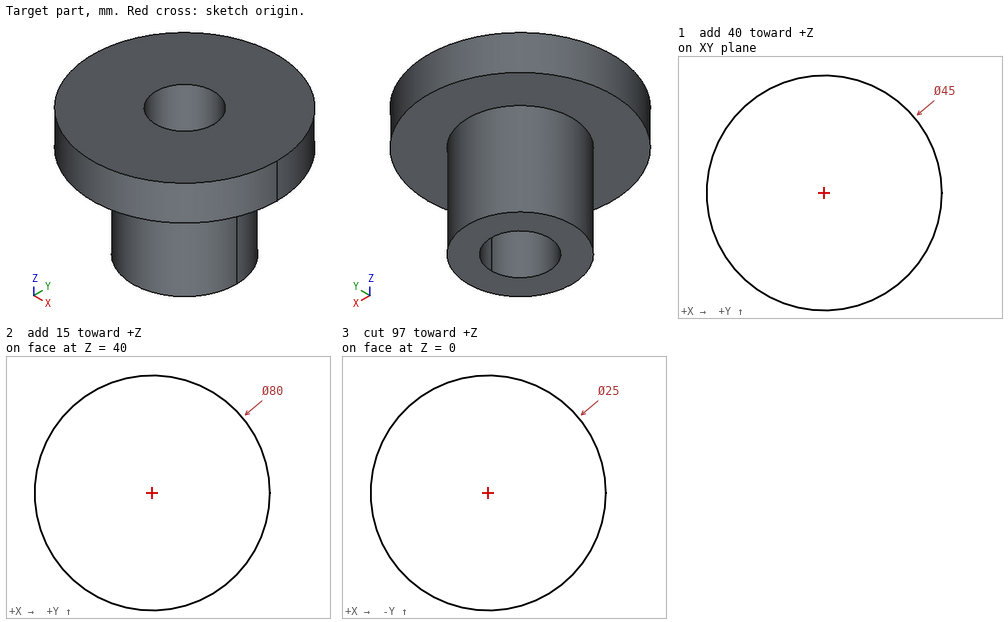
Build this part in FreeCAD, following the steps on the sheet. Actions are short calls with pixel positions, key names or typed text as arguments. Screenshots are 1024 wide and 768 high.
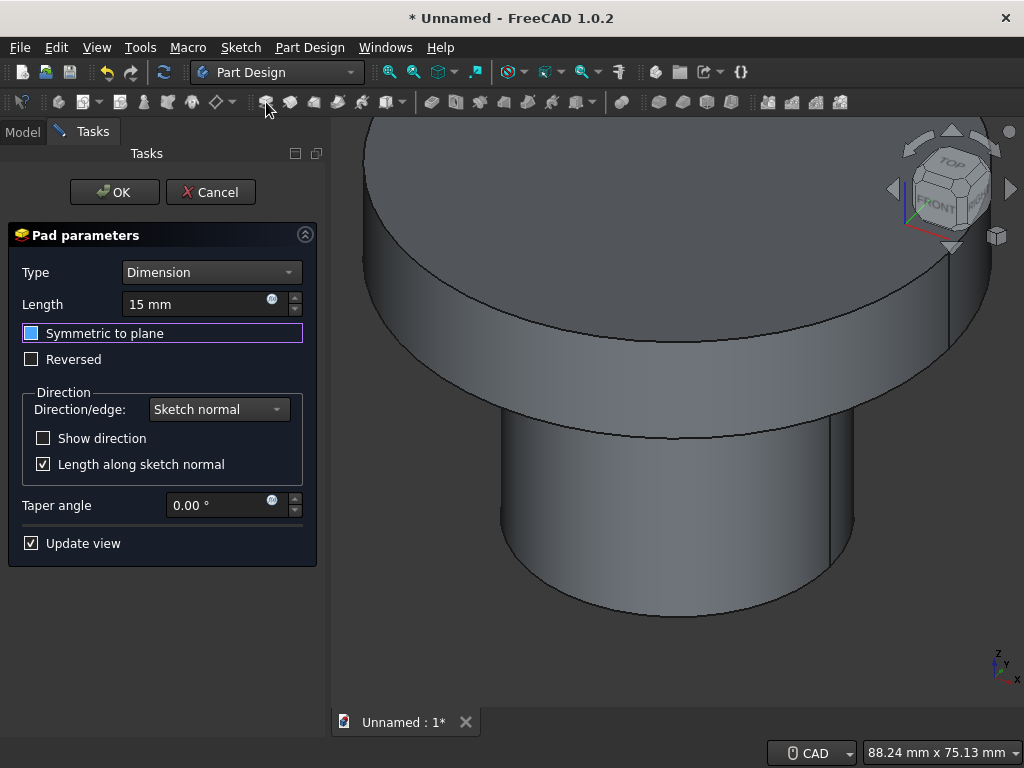
click(115, 192)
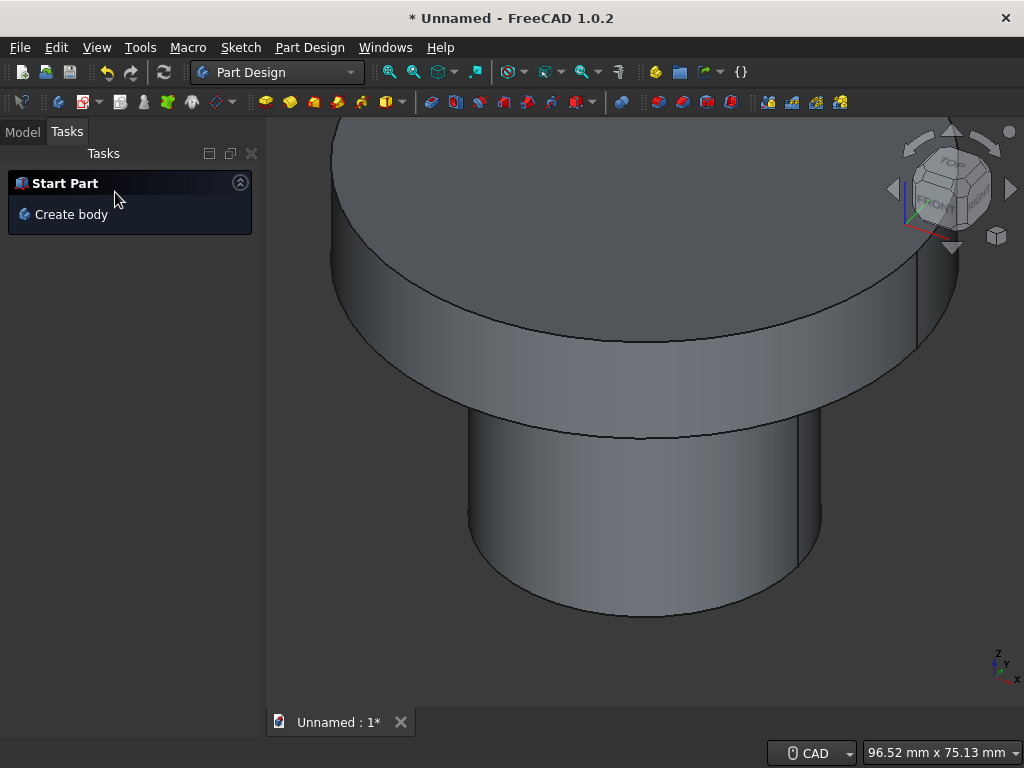
click(390, 72)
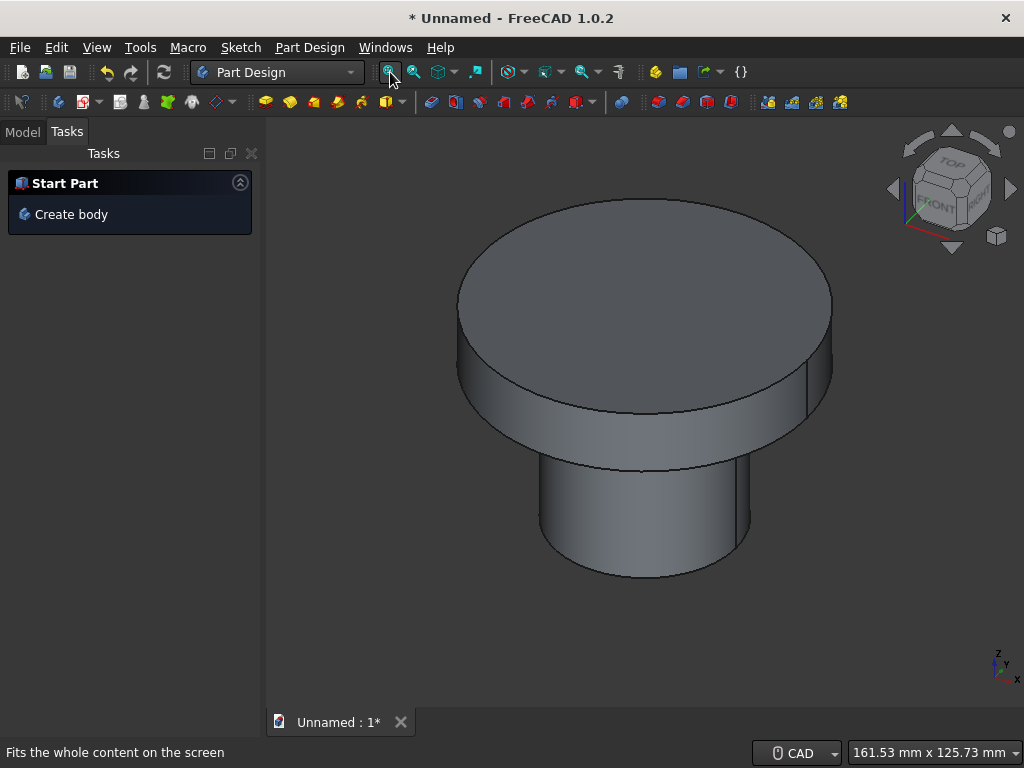
key(5)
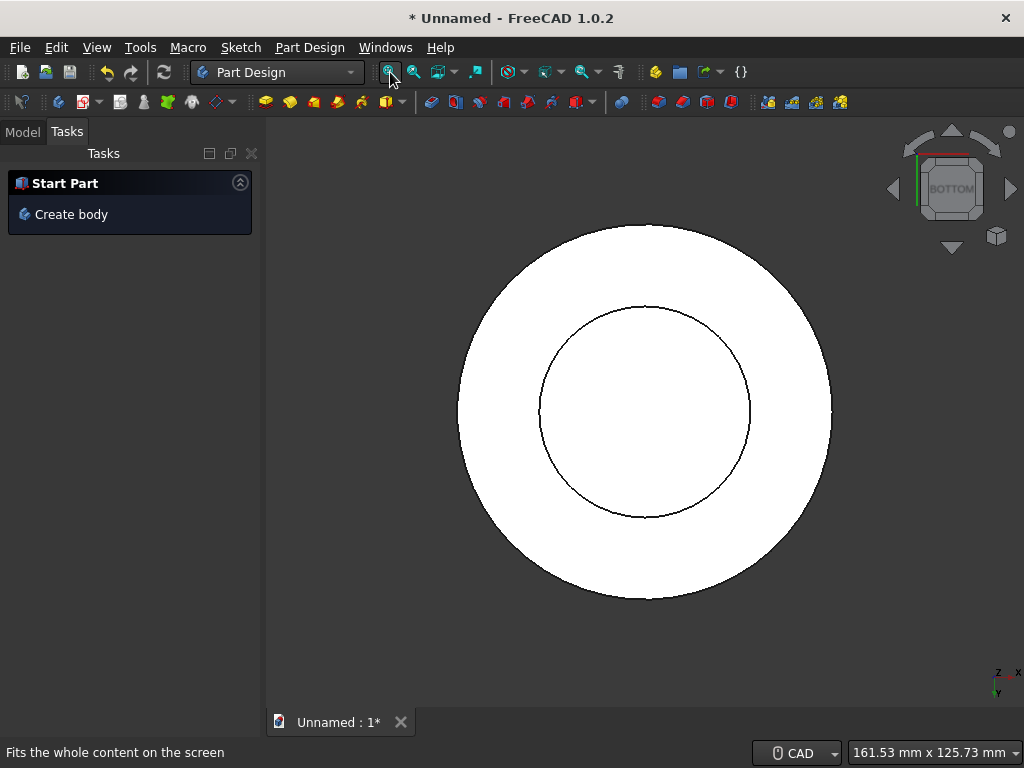
click(645, 411)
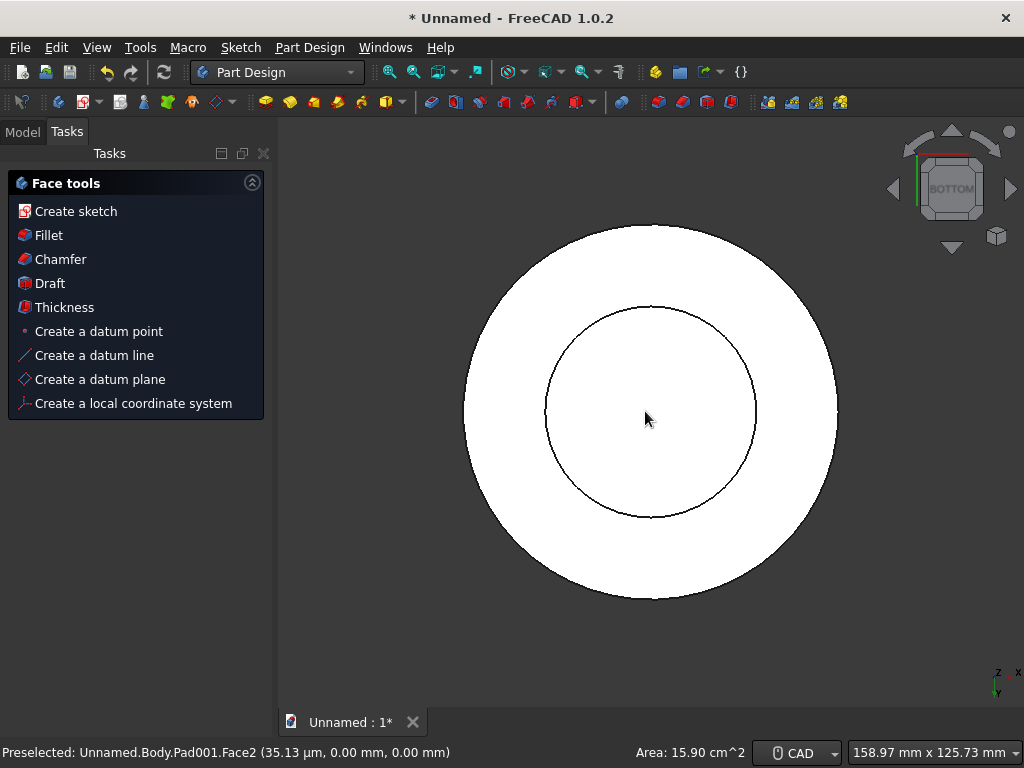
click(84, 102)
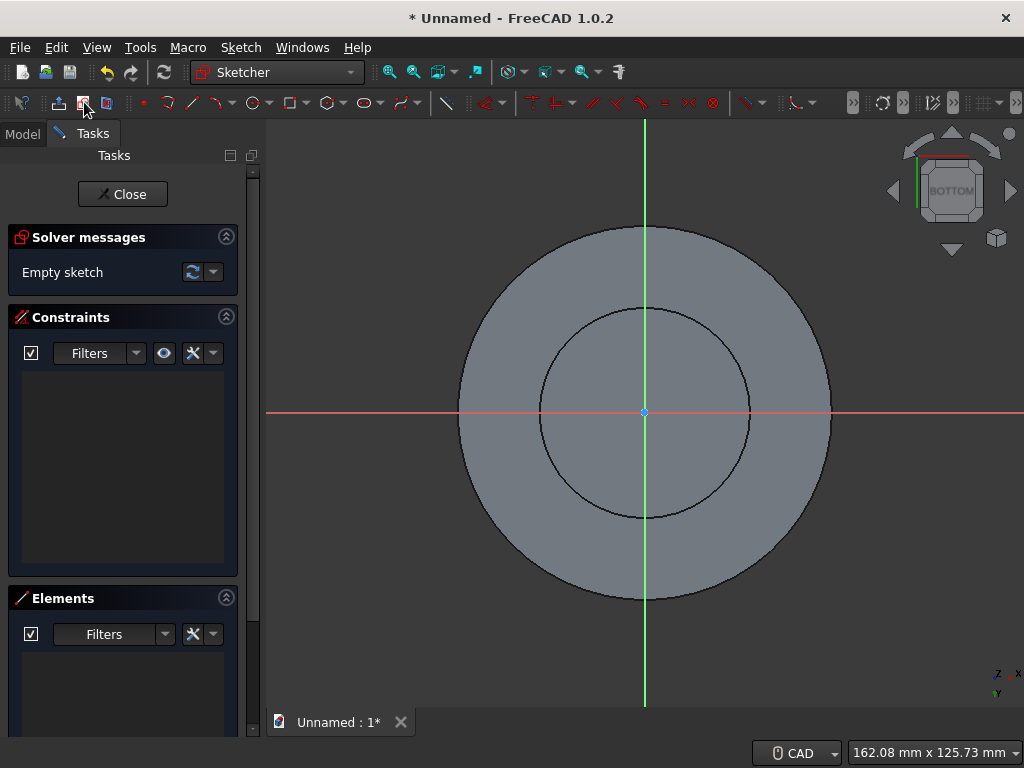
scroll(674, 413, up, 6)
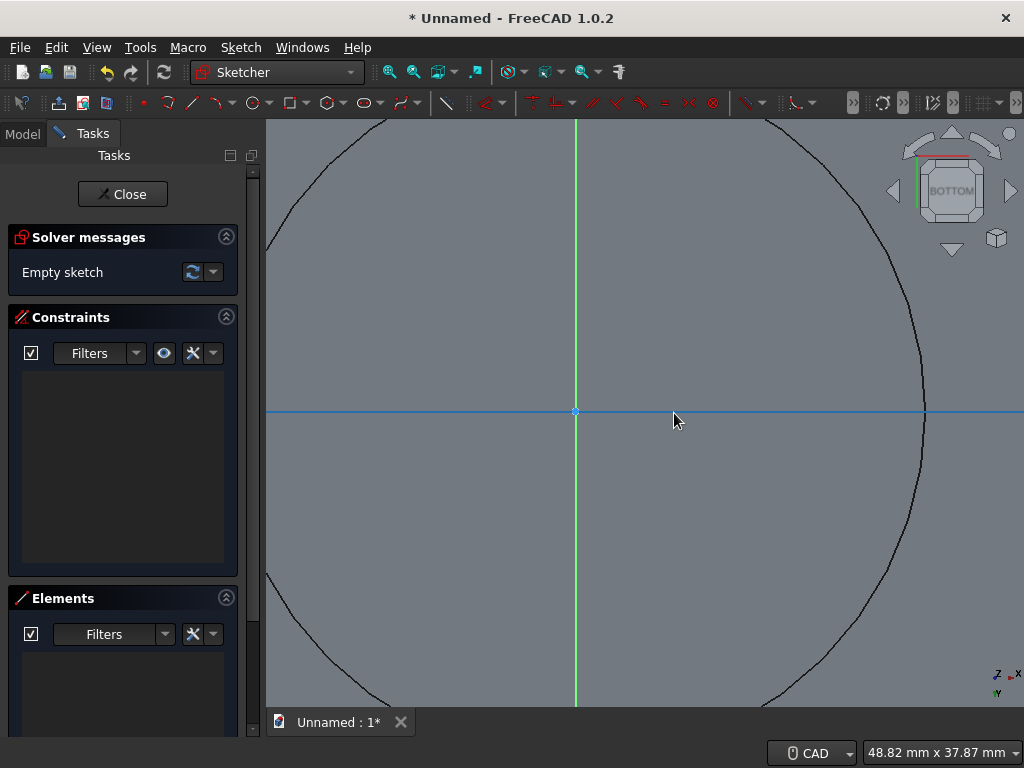
click(254, 104)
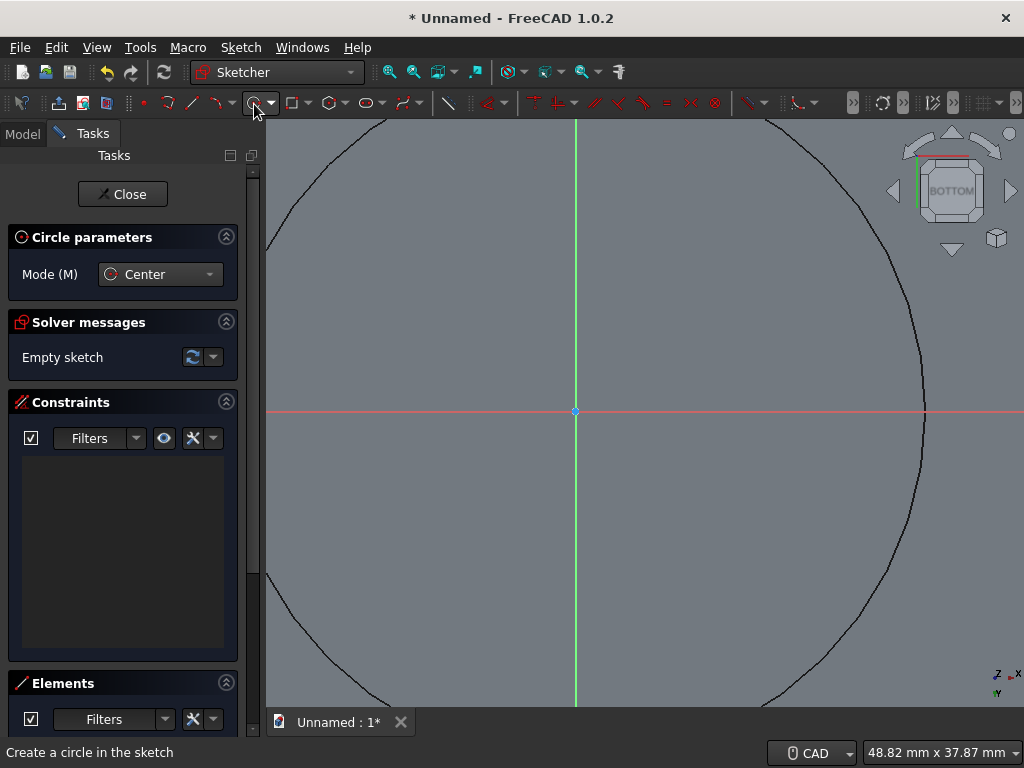
click(576, 412)
click(713, 275)
key(Escape)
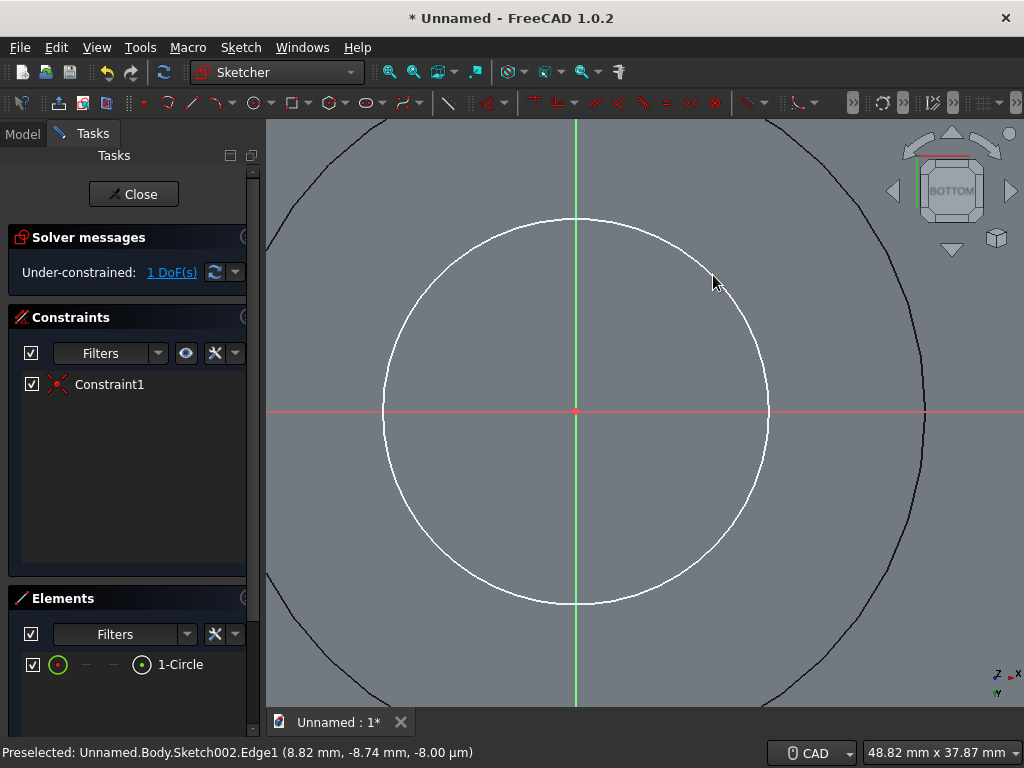
click(488, 104)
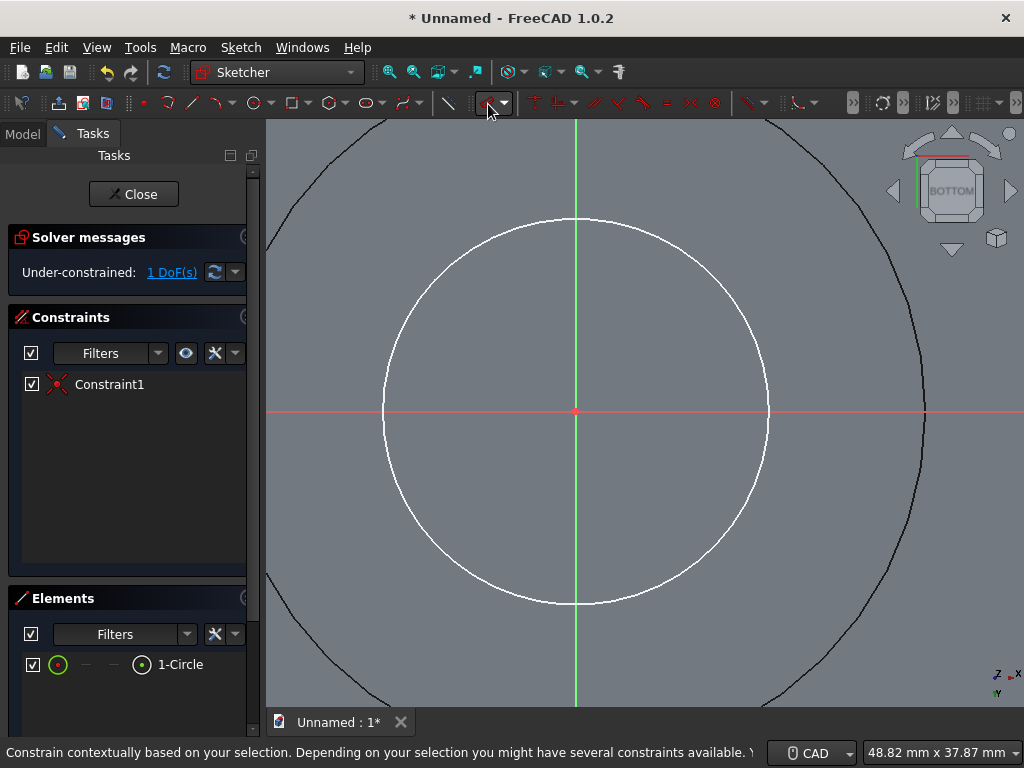
click(712, 275)
click(735, 252)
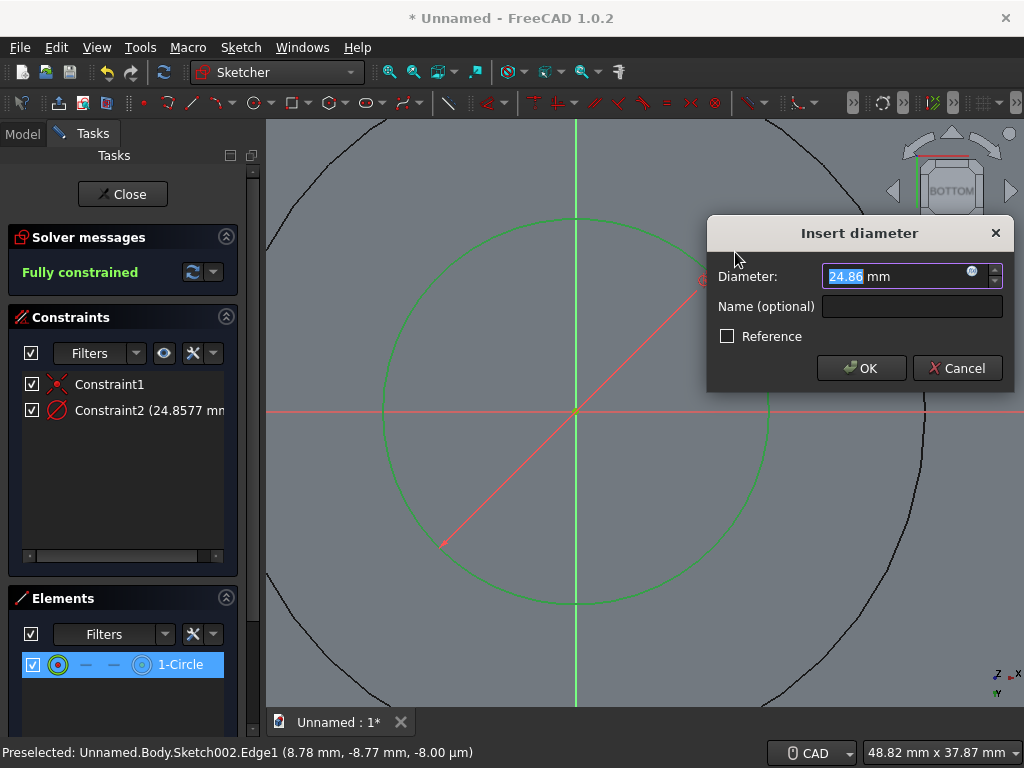
text(25)
key(Return)
key(Escape)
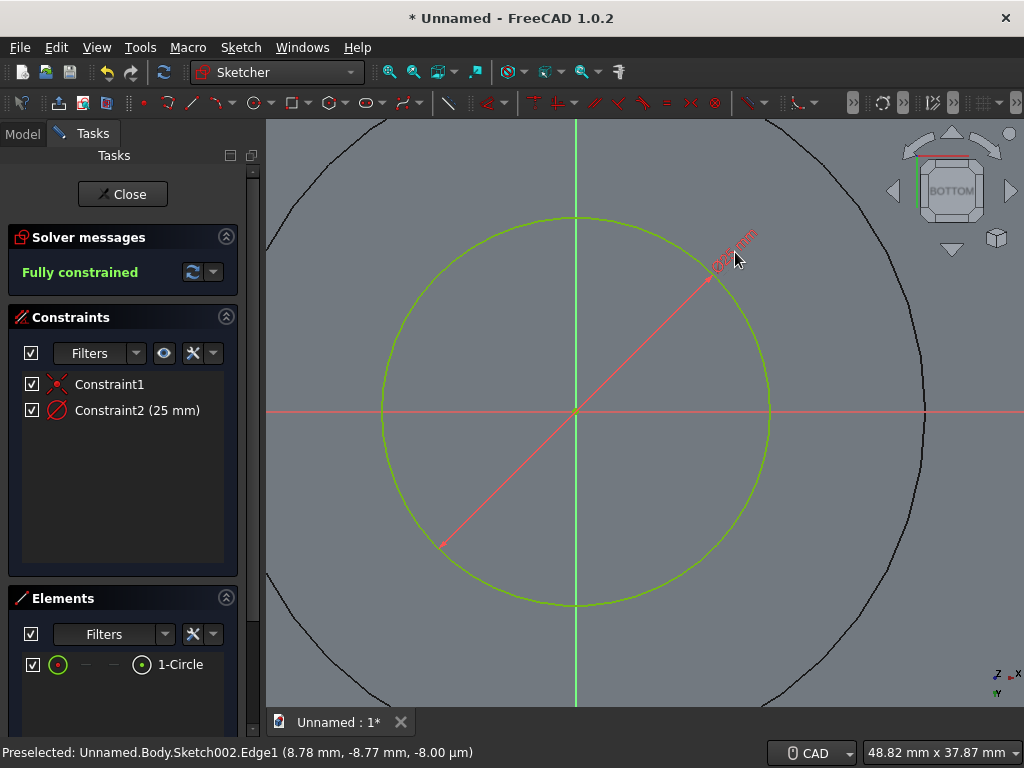
click(123, 194)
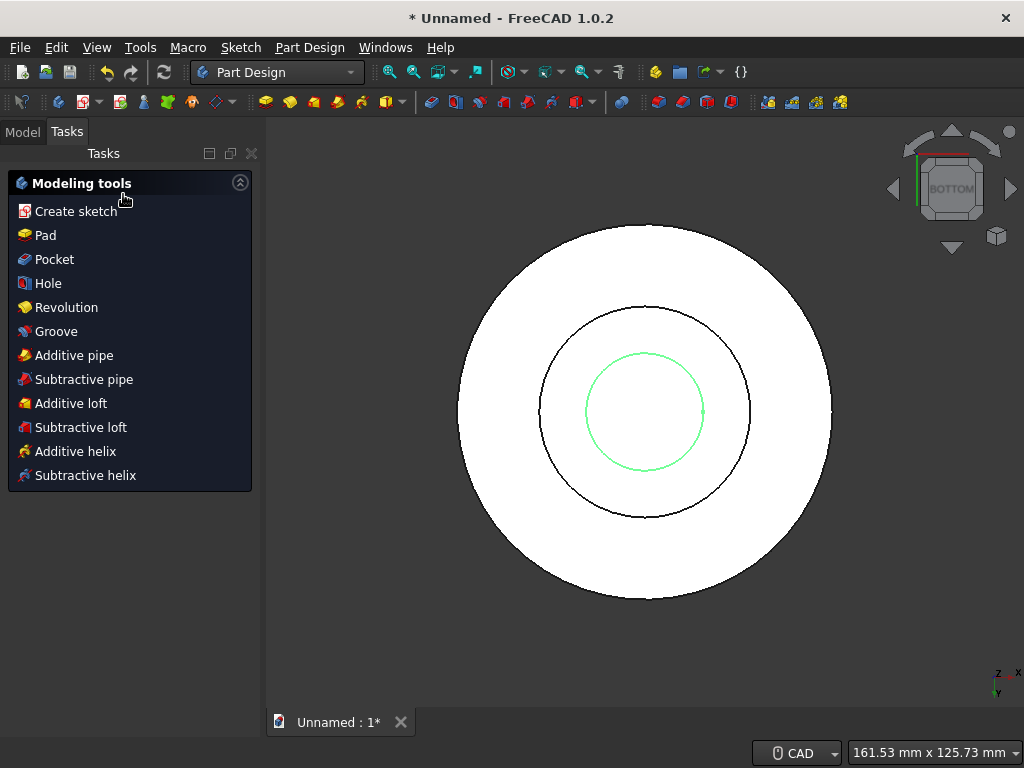
click(432, 102)